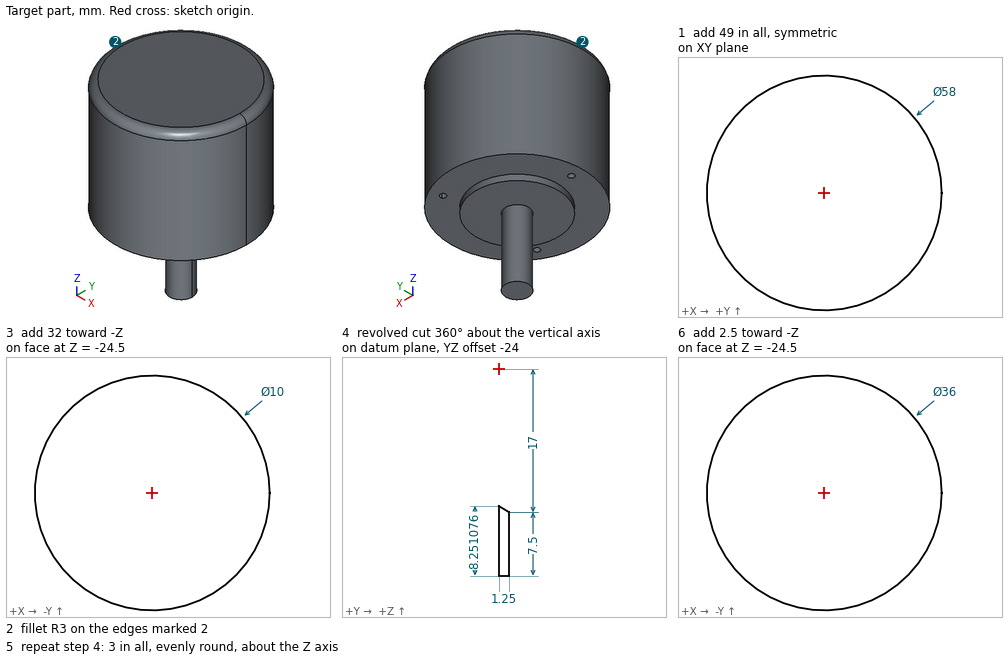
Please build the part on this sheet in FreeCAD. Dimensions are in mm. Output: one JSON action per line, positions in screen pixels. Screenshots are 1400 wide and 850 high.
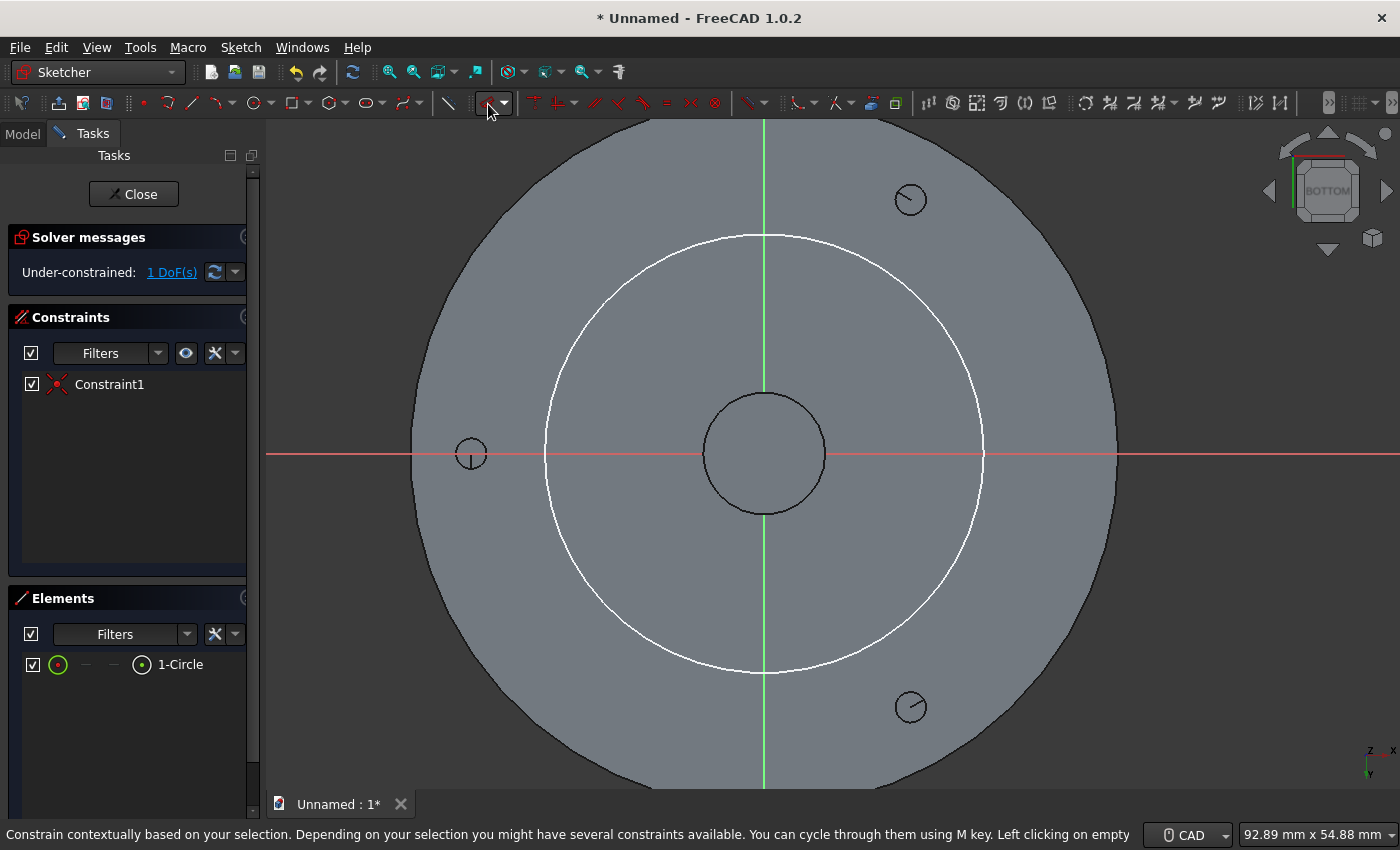
{"action": "left_click", "coordinate": [919, 298]}
{"action": "left_click", "coordinate": [942, 275]}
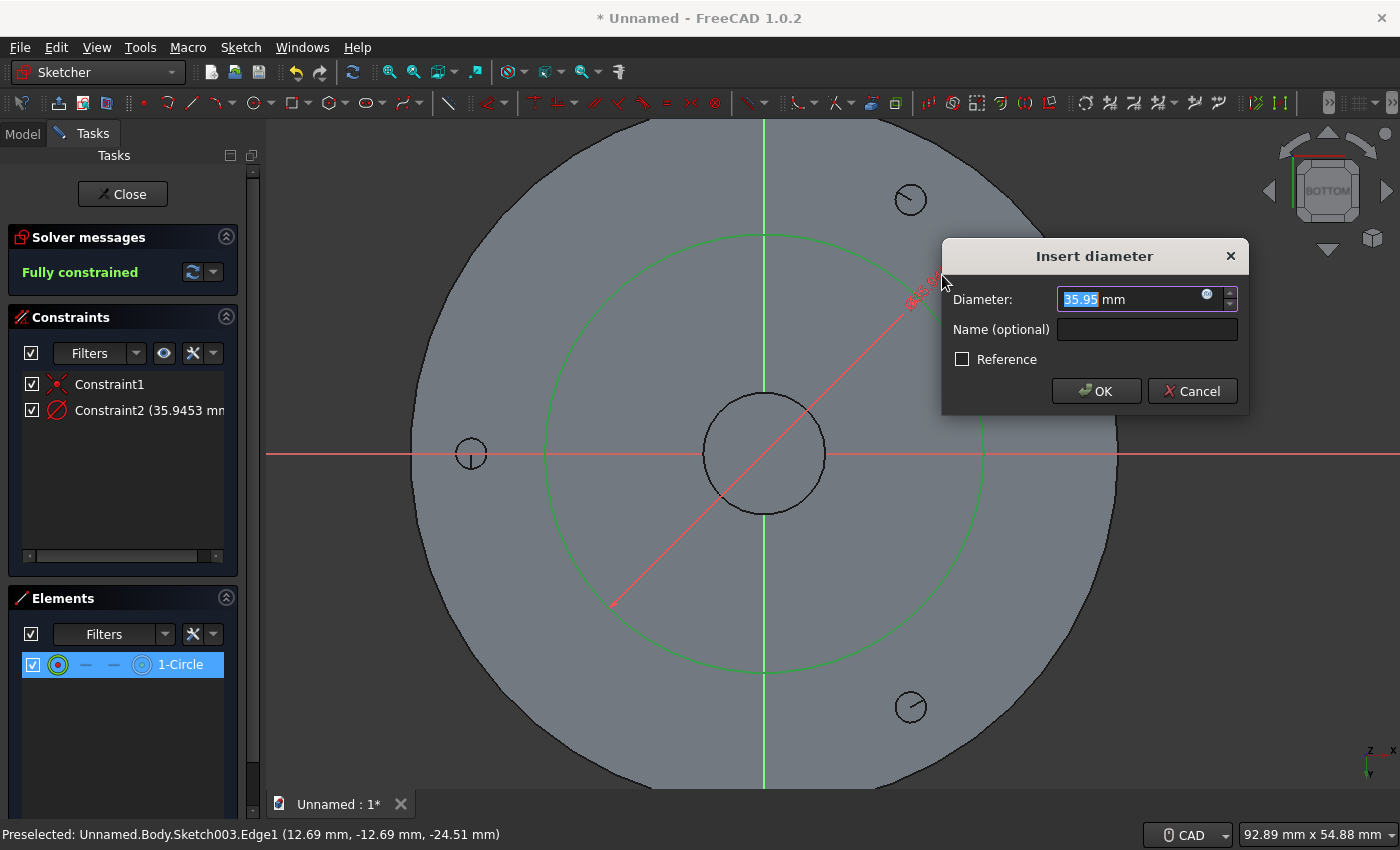
{"action": "type", "text": "36"}
{"action": "key", "text": "Return"}
{"action": "key", "text": "Escape"}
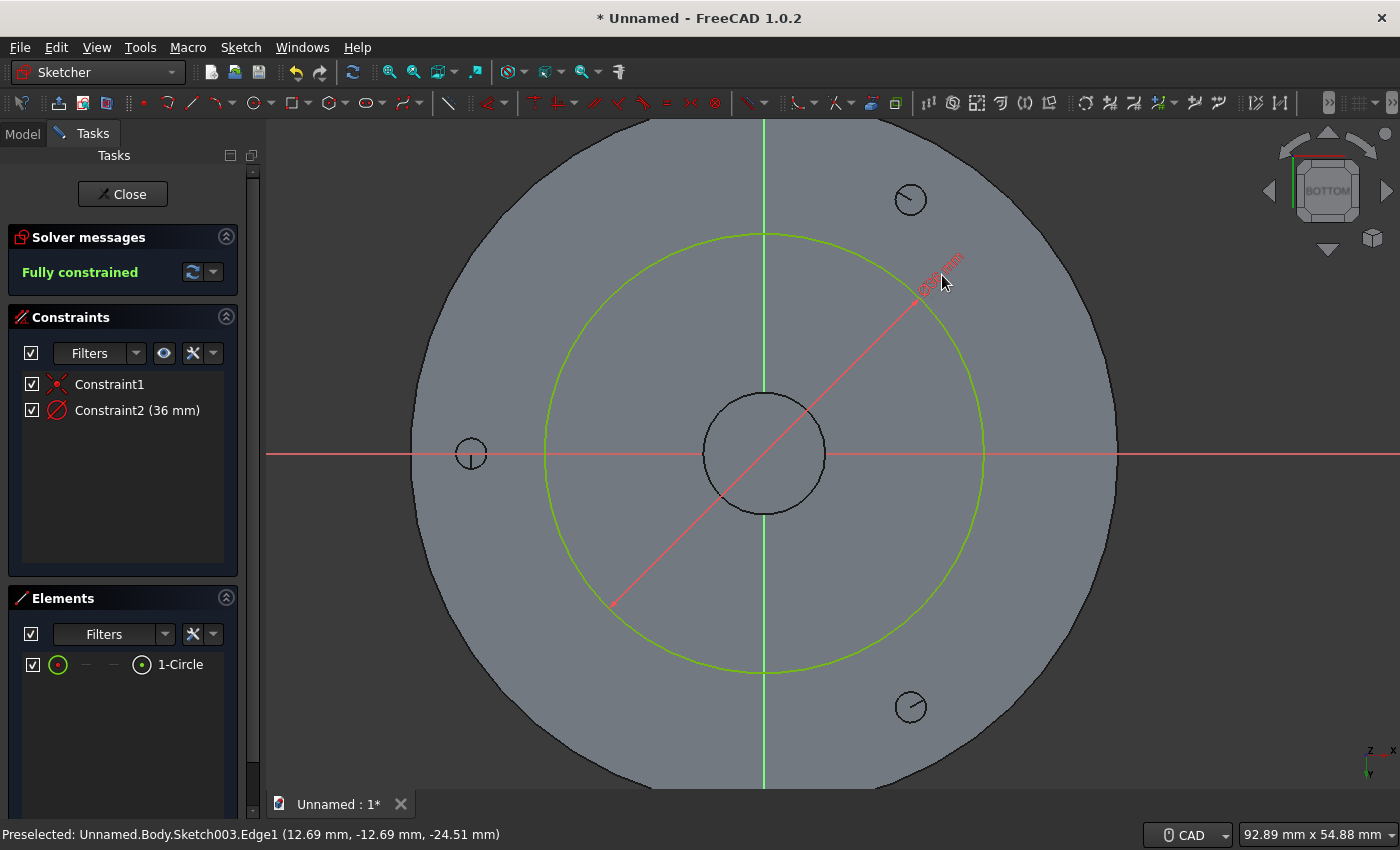
{"action": "left_click", "coordinate": [123, 194]}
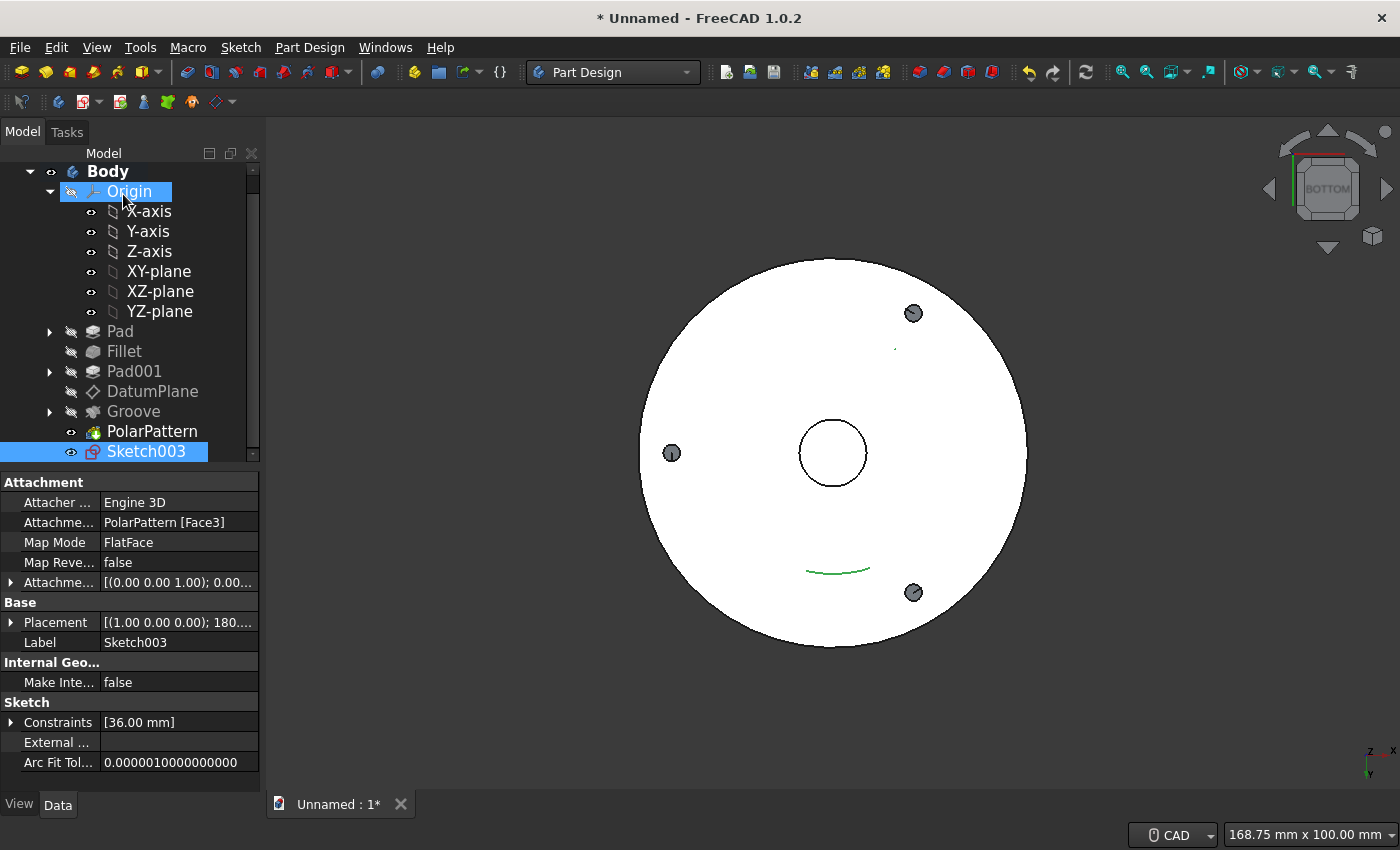
{"action": "left_click", "coordinate": [22, 72]}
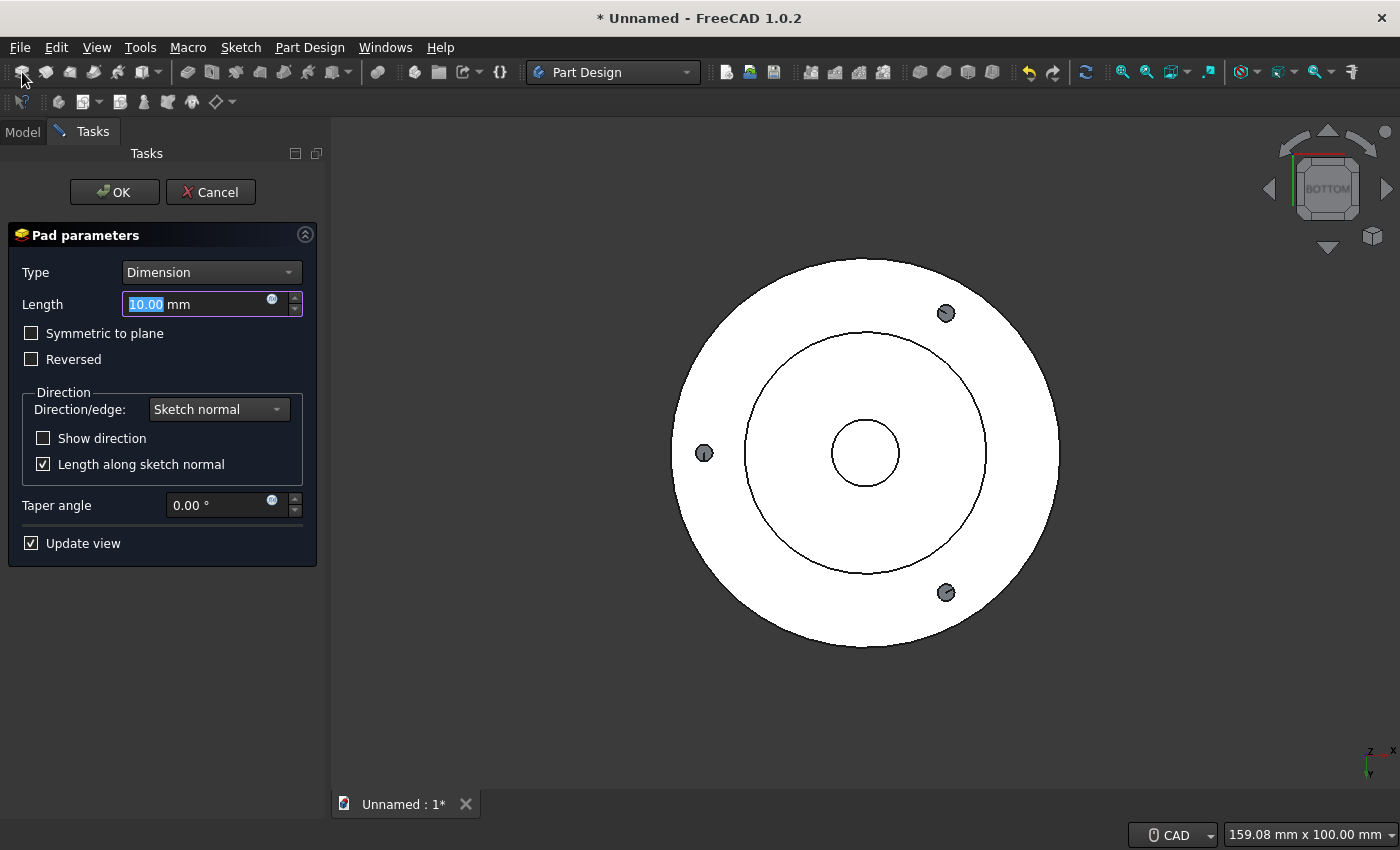
{"action": "type", "text": "2.5"}
{"action": "key", "text": "Tab"}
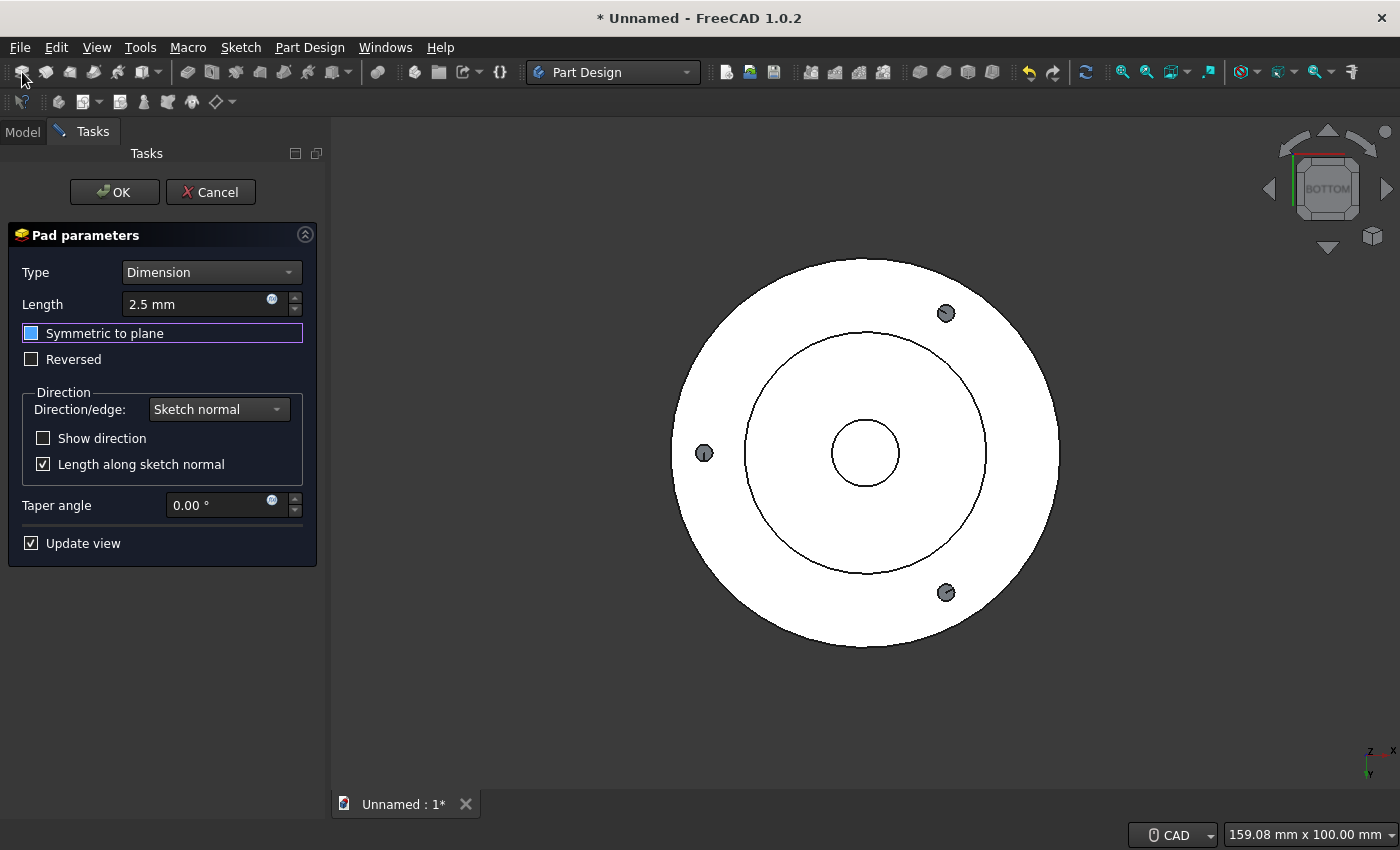
{"action": "left_click", "coordinate": [115, 192]}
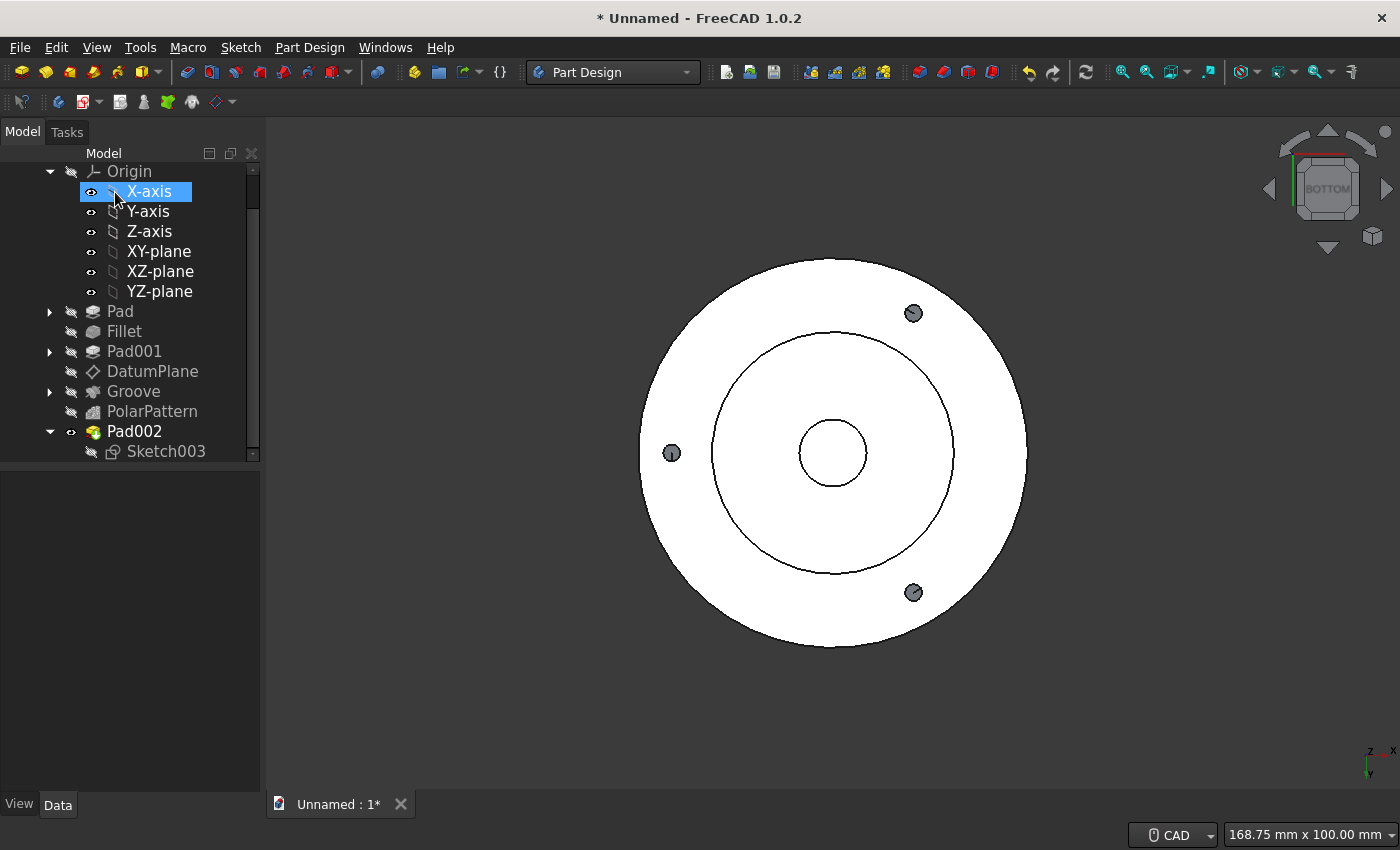
{"action": "key", "text": "0"}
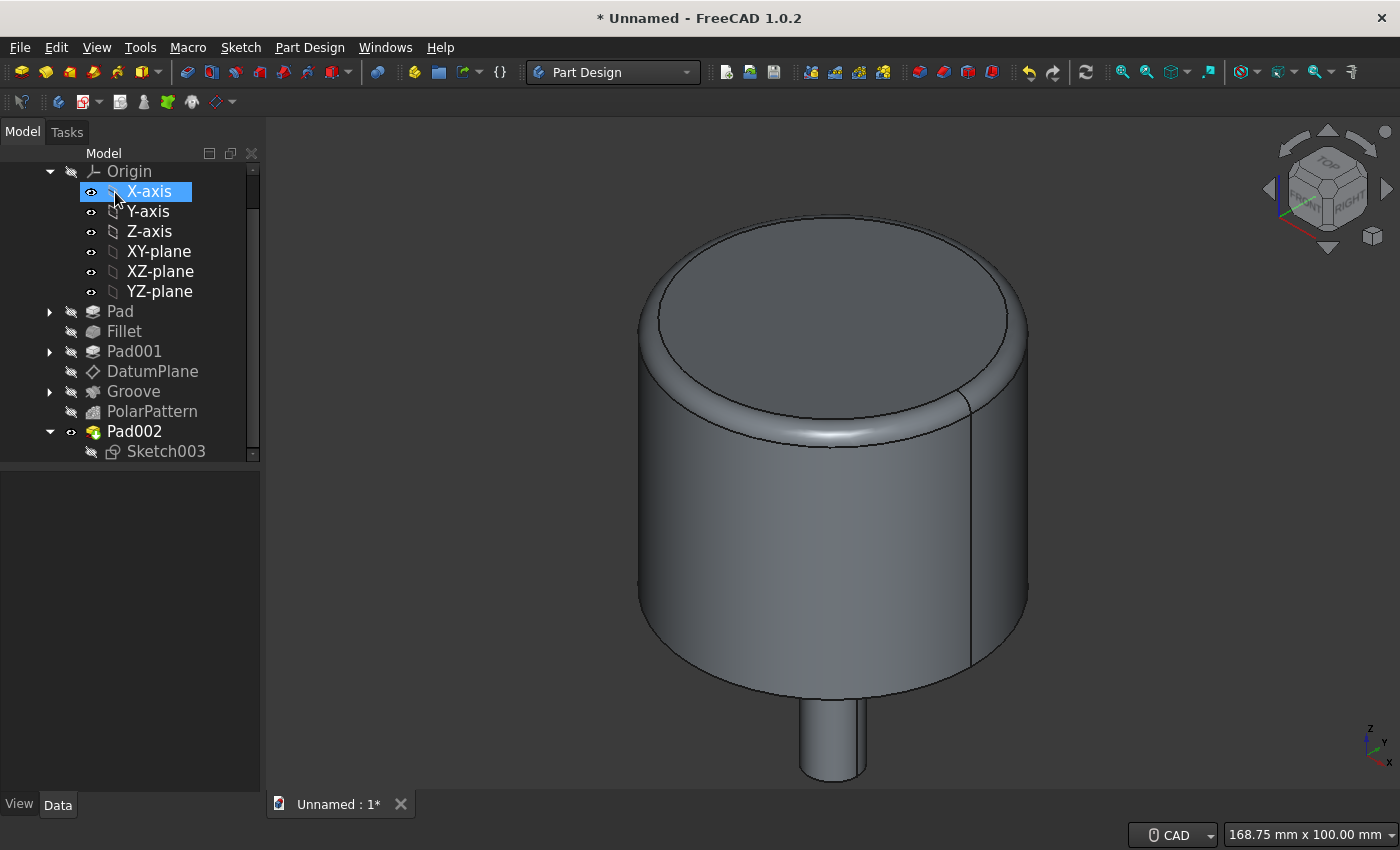
{"action": "left_click", "coordinate": [1124, 72]}